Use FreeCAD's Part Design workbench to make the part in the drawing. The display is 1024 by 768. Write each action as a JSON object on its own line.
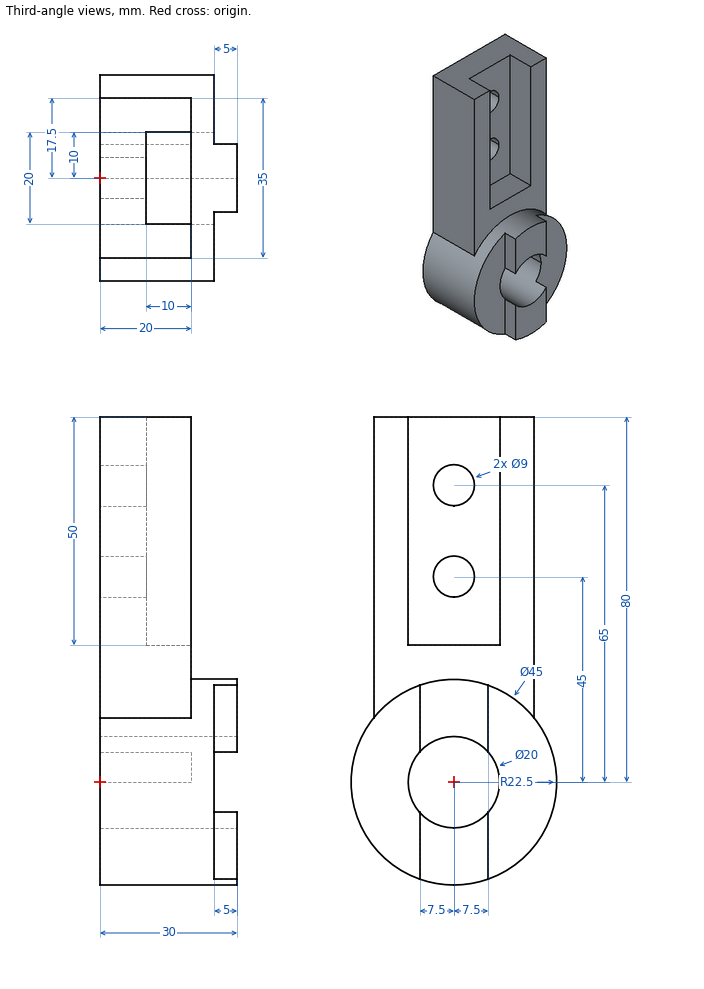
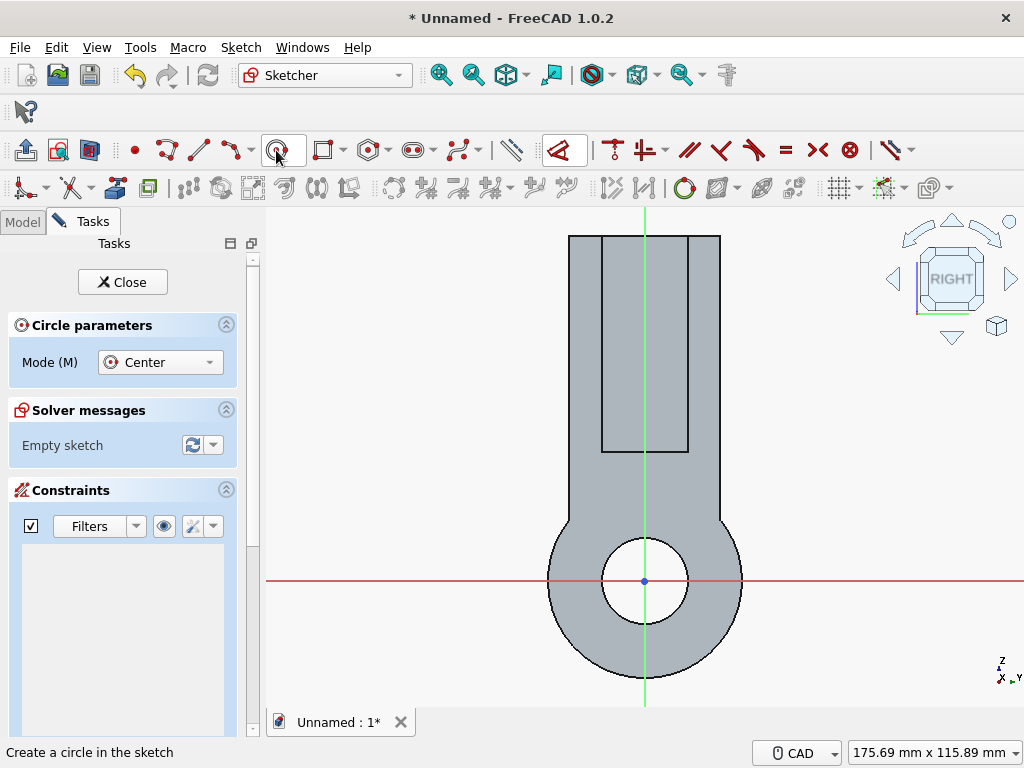
{"action": "left_click", "coordinate": [645, 301]}
{"action": "mouse_move", "coordinate": [663, 294]}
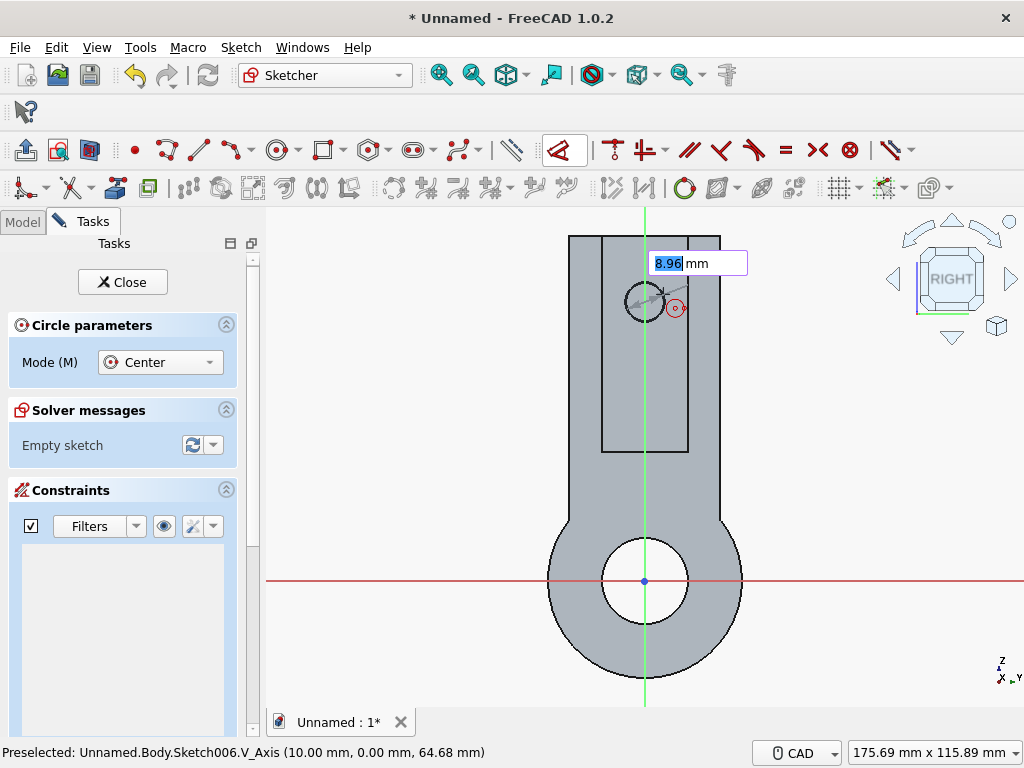
{"action": "type", "text": "9"}
{"action": "key", "text": "Return"}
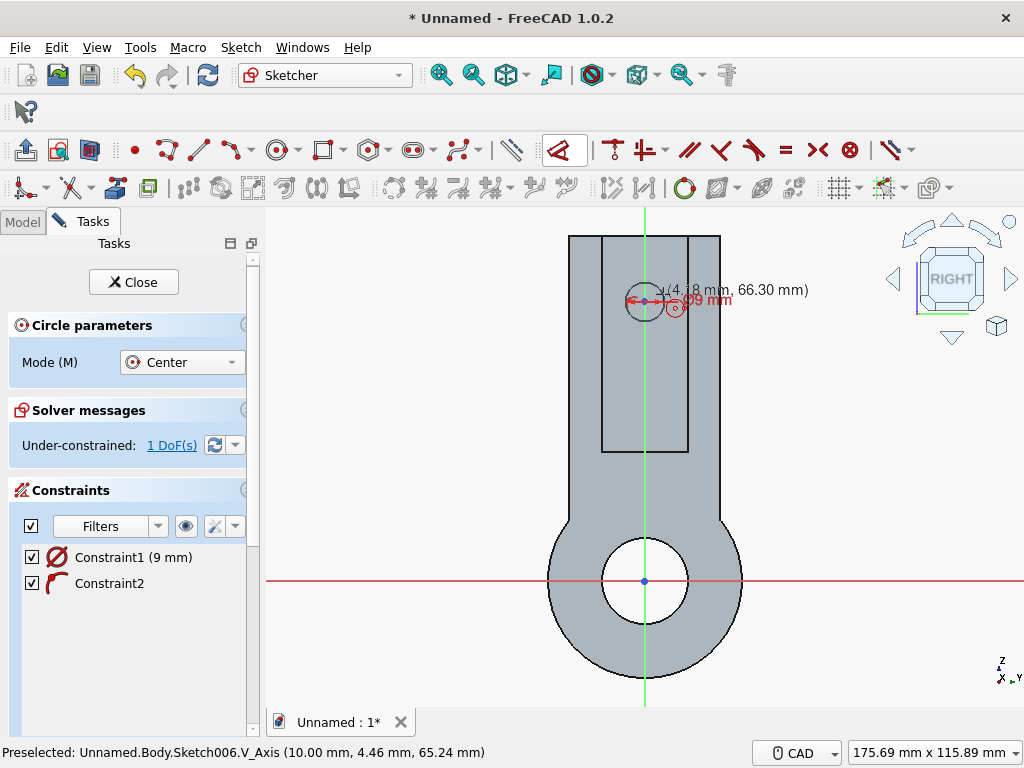
{"action": "left_click", "coordinate": [645, 387]}
{"action": "mouse_move", "coordinate": [663, 380]}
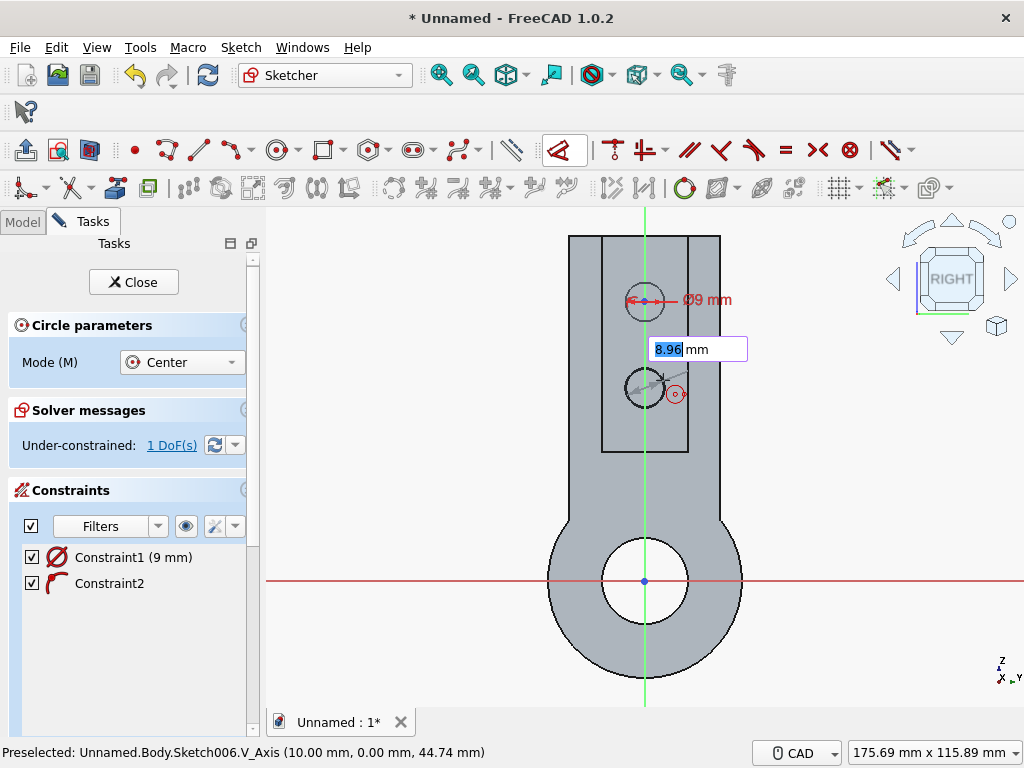
{"action": "type", "text": "9"}
{"action": "key", "text": "Return"}
{"action": "key", "text": "Escape"}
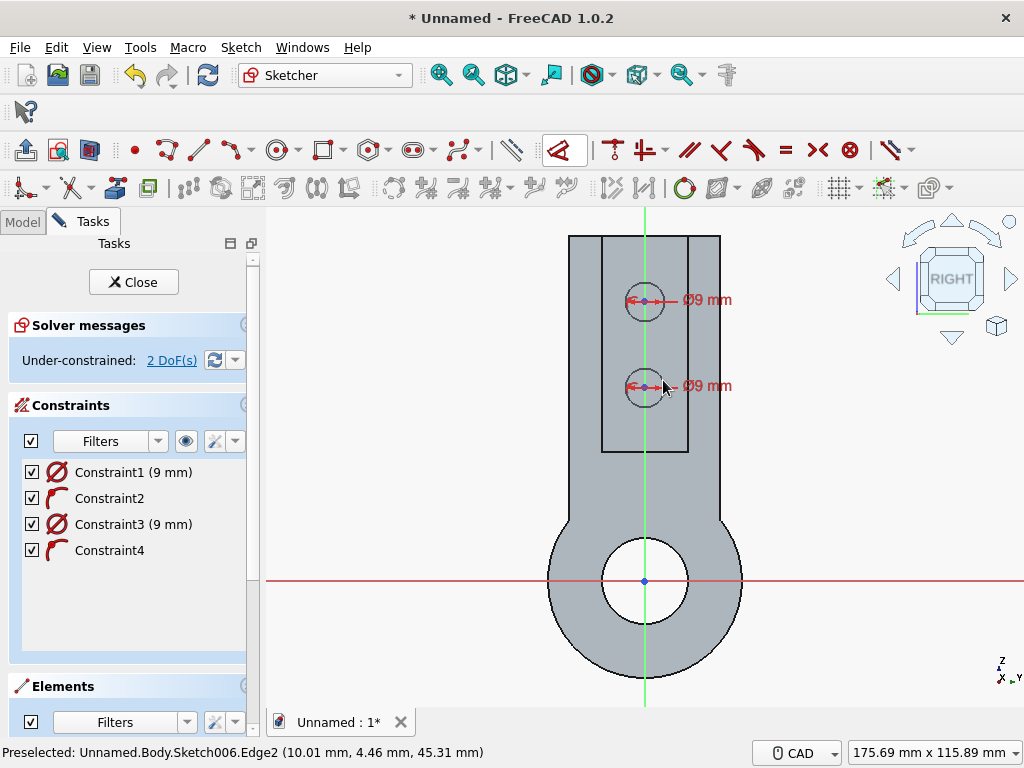
{"action": "left_click", "coordinate": [645, 302]}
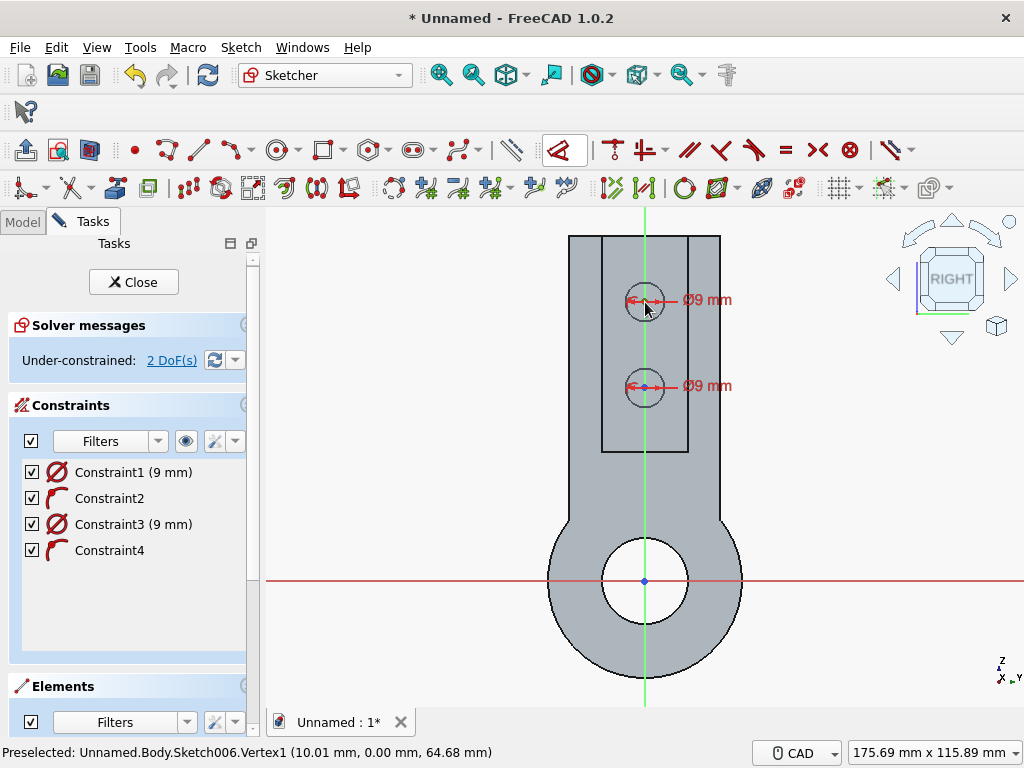
{"action": "left_click", "coordinate": [582, 150]}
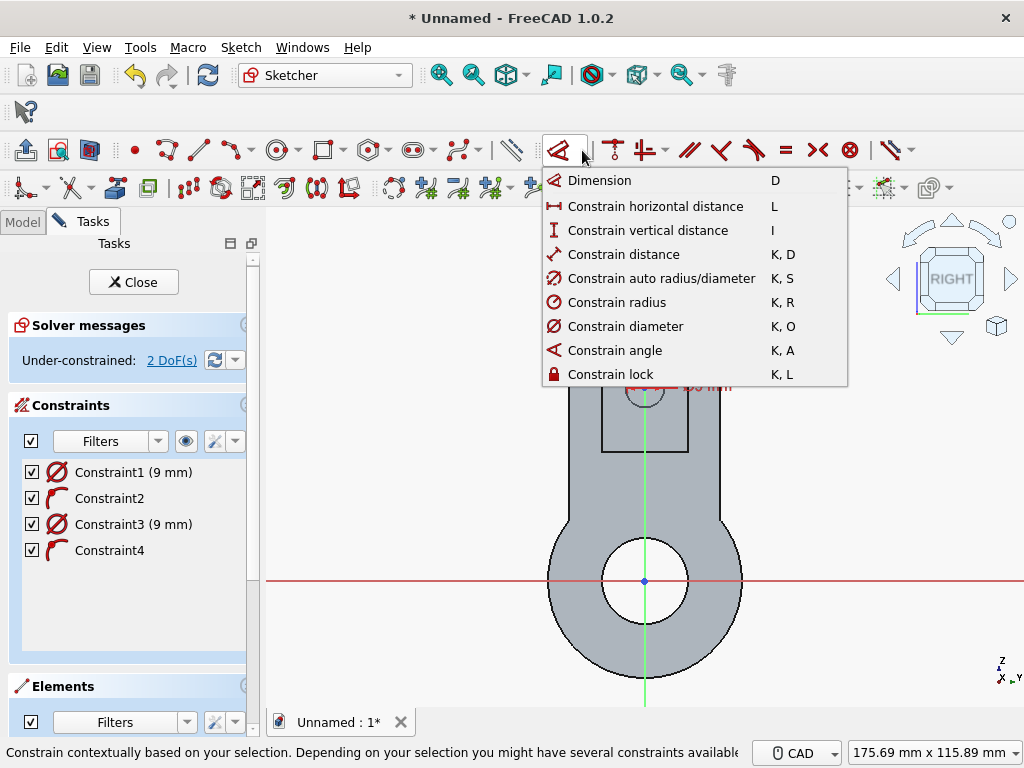
{"action": "left_click", "coordinate": [695, 230]}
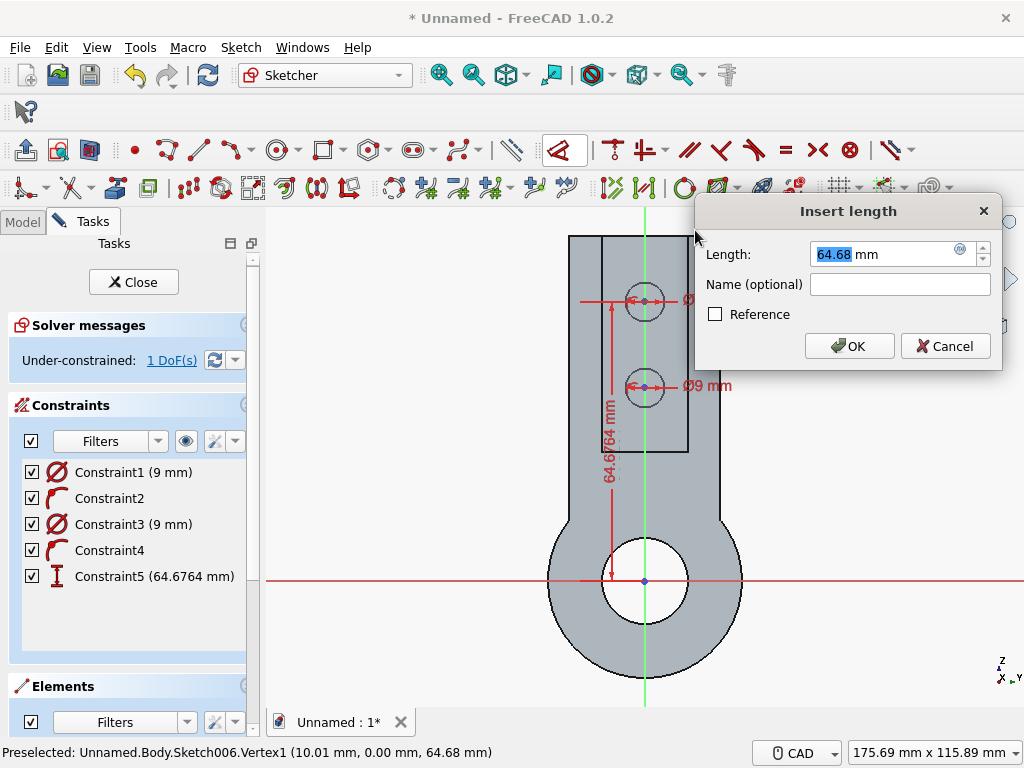
{"action": "type", "text": "65"}
{"action": "key", "text": "Return"}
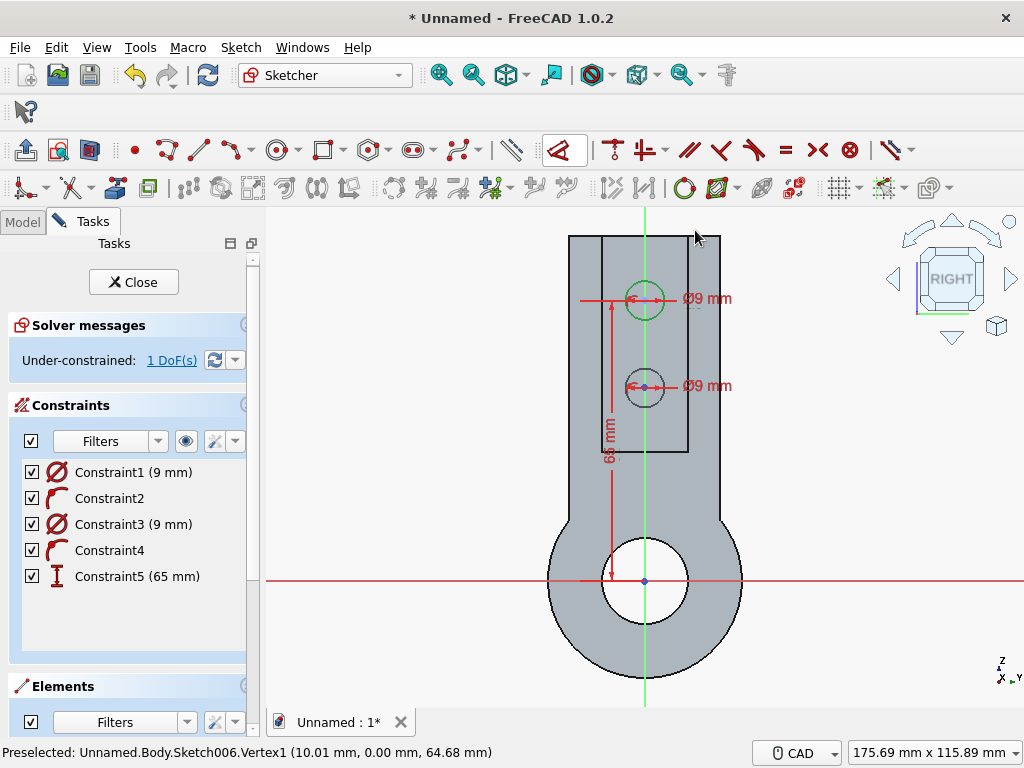
{"action": "left_click", "coordinate": [645, 388]}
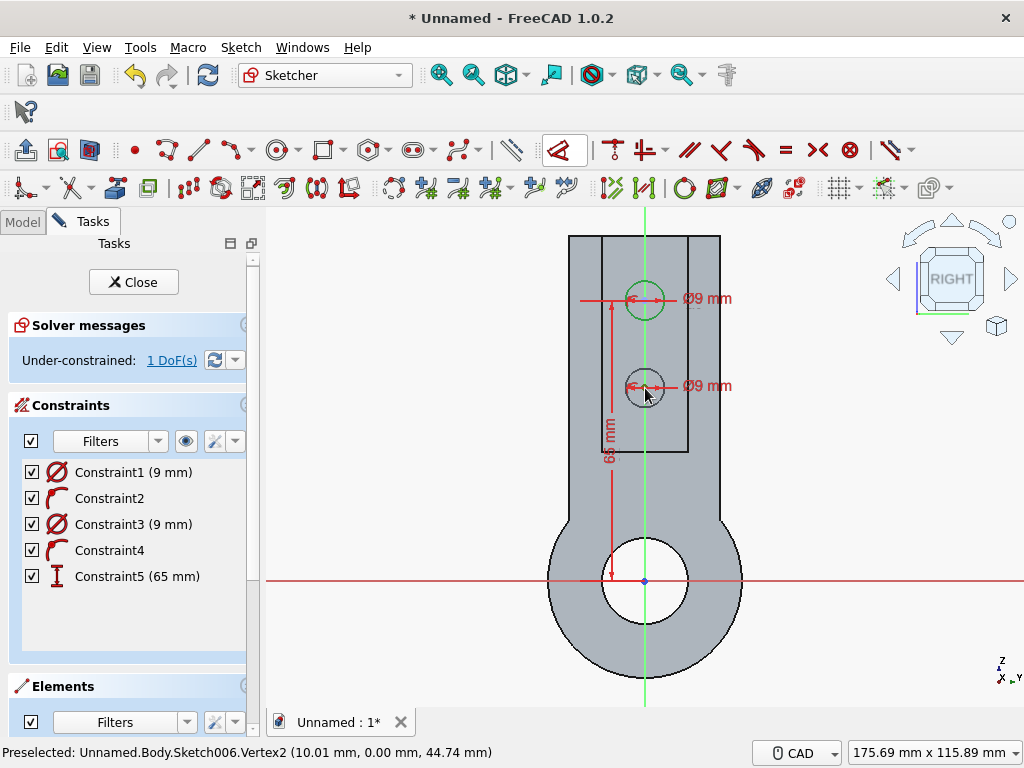
{"action": "left_click", "coordinate": [582, 150]}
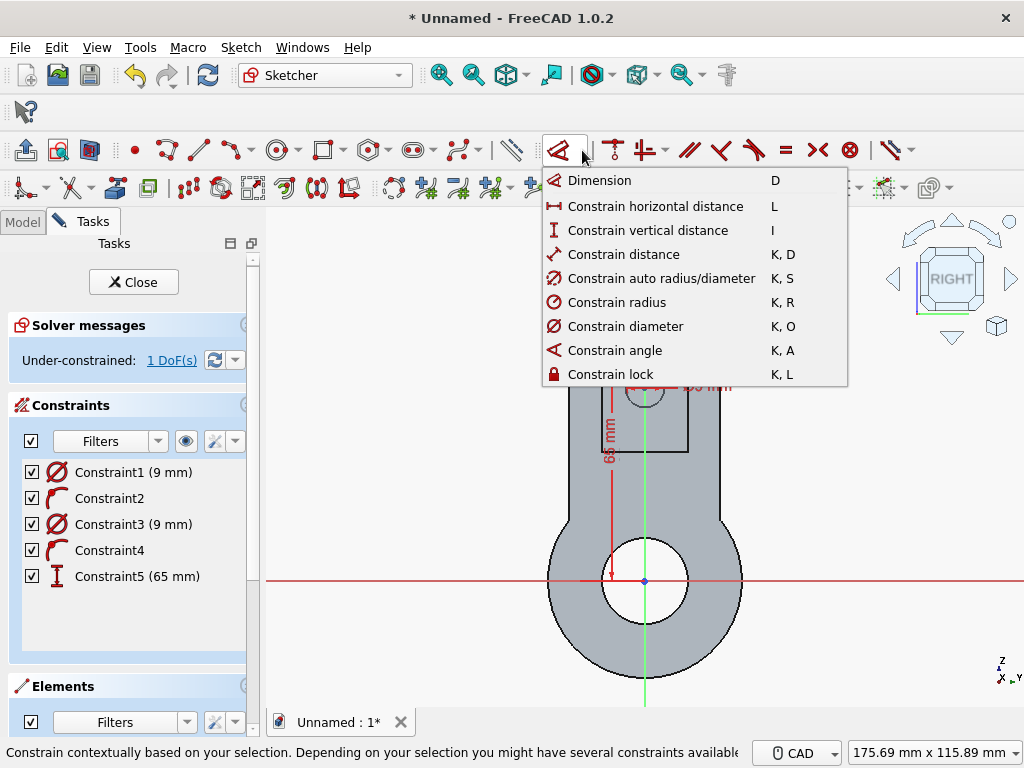
{"action": "left_click", "coordinate": [695, 230]}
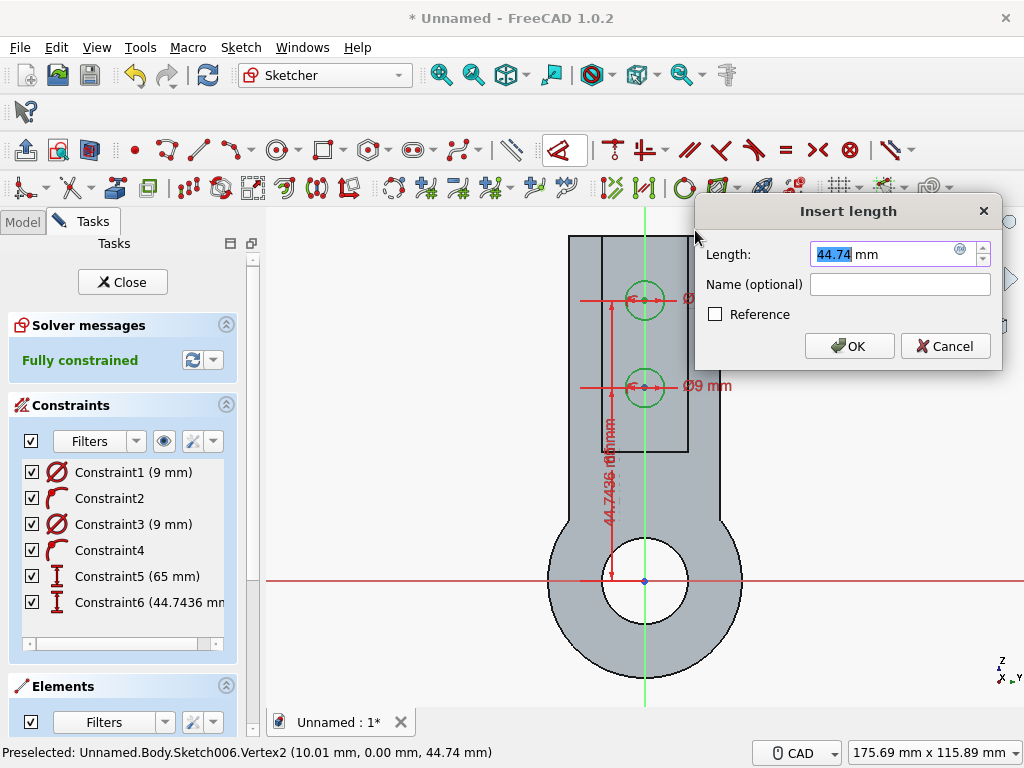
{"action": "type", "text": "45"}
{"action": "key", "text": "Return"}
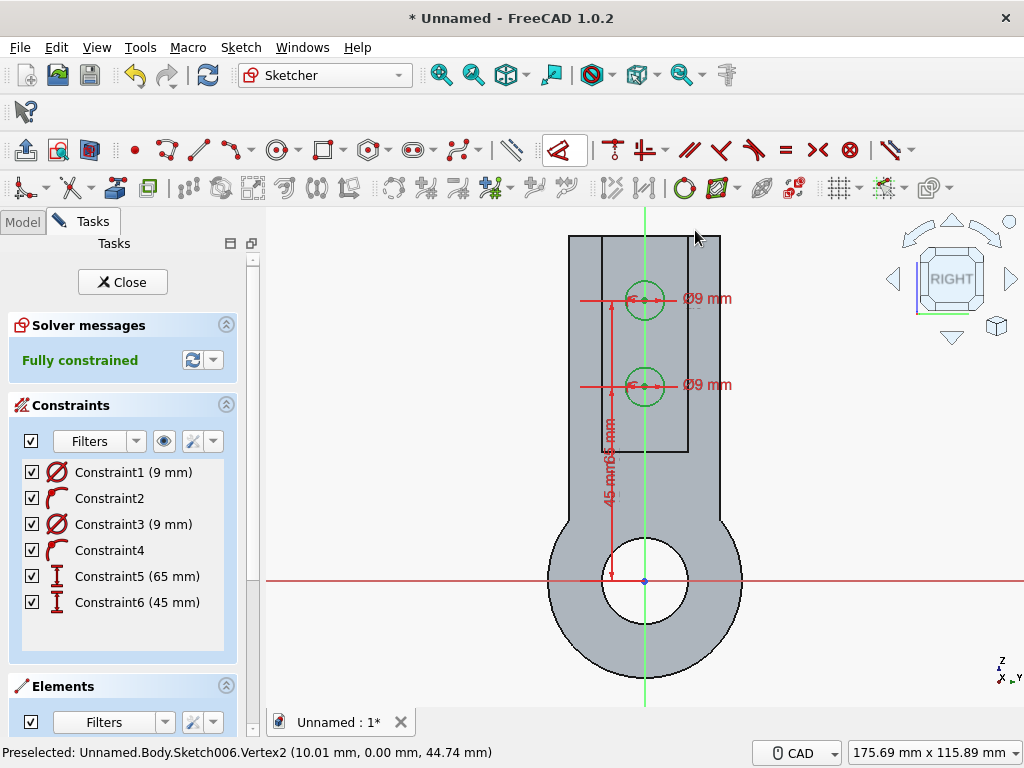
{"action": "left_click", "coordinate": [123, 282]}